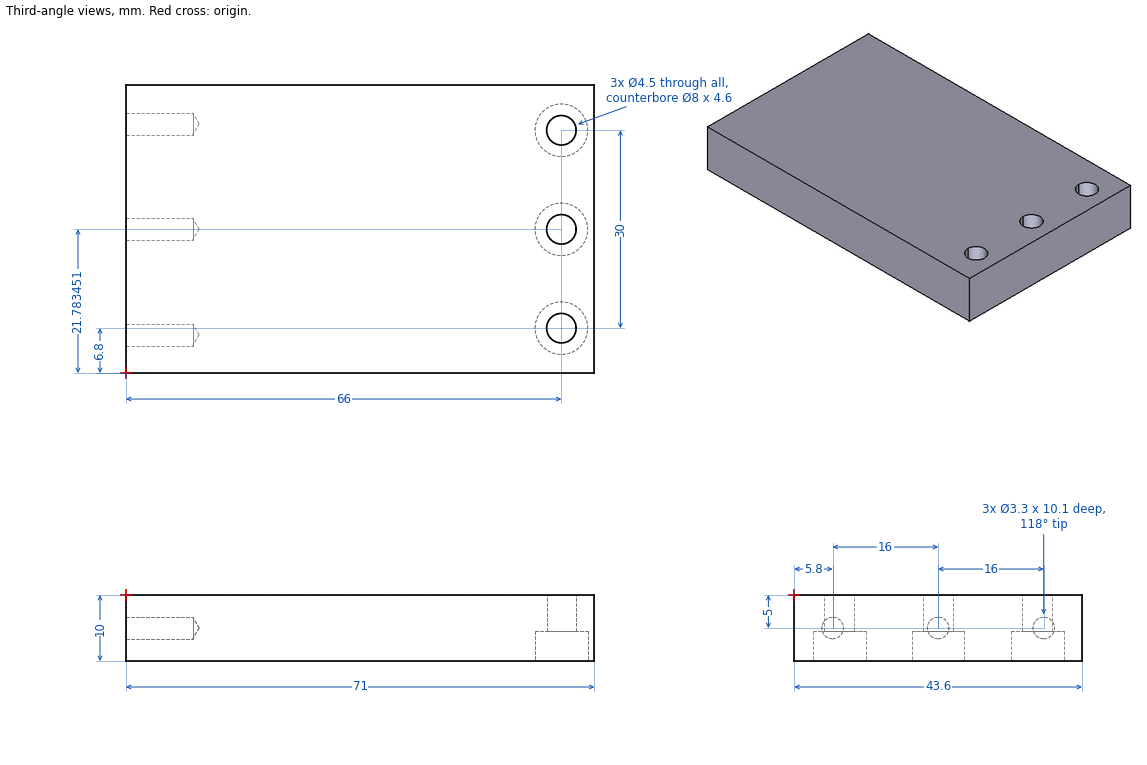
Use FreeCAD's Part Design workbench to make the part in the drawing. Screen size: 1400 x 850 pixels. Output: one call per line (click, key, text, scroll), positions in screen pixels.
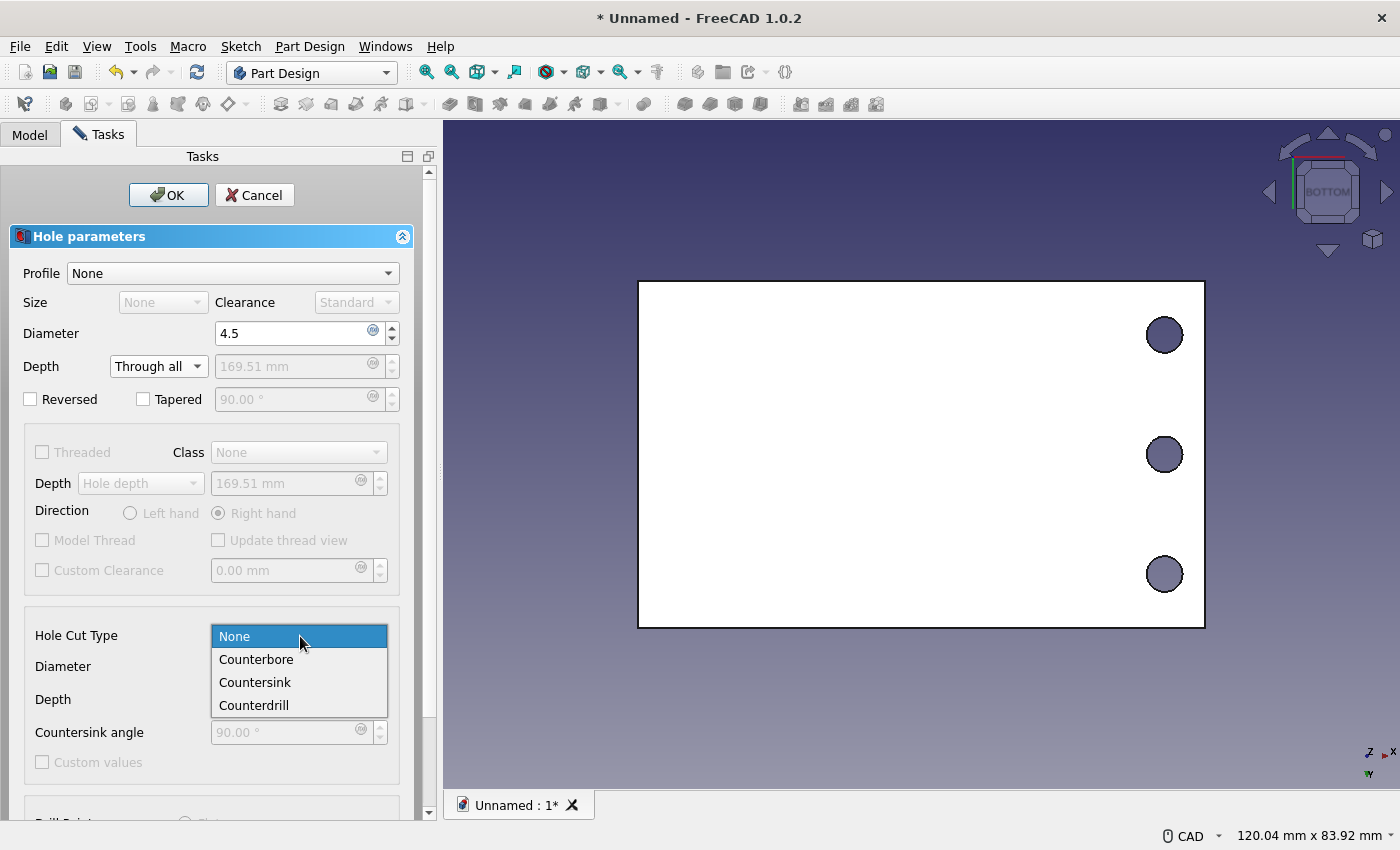
click(298, 660)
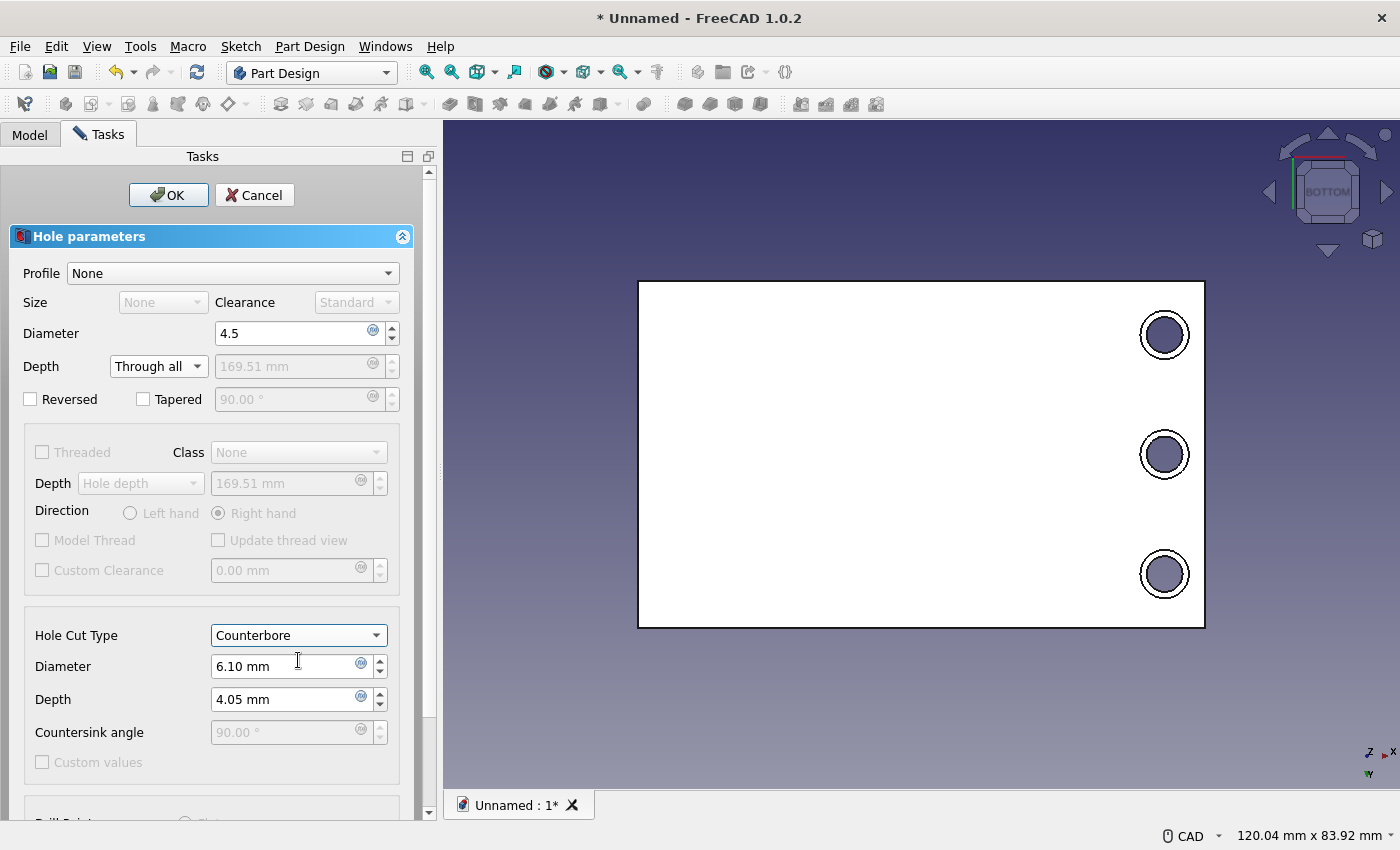
triple_click(292, 666)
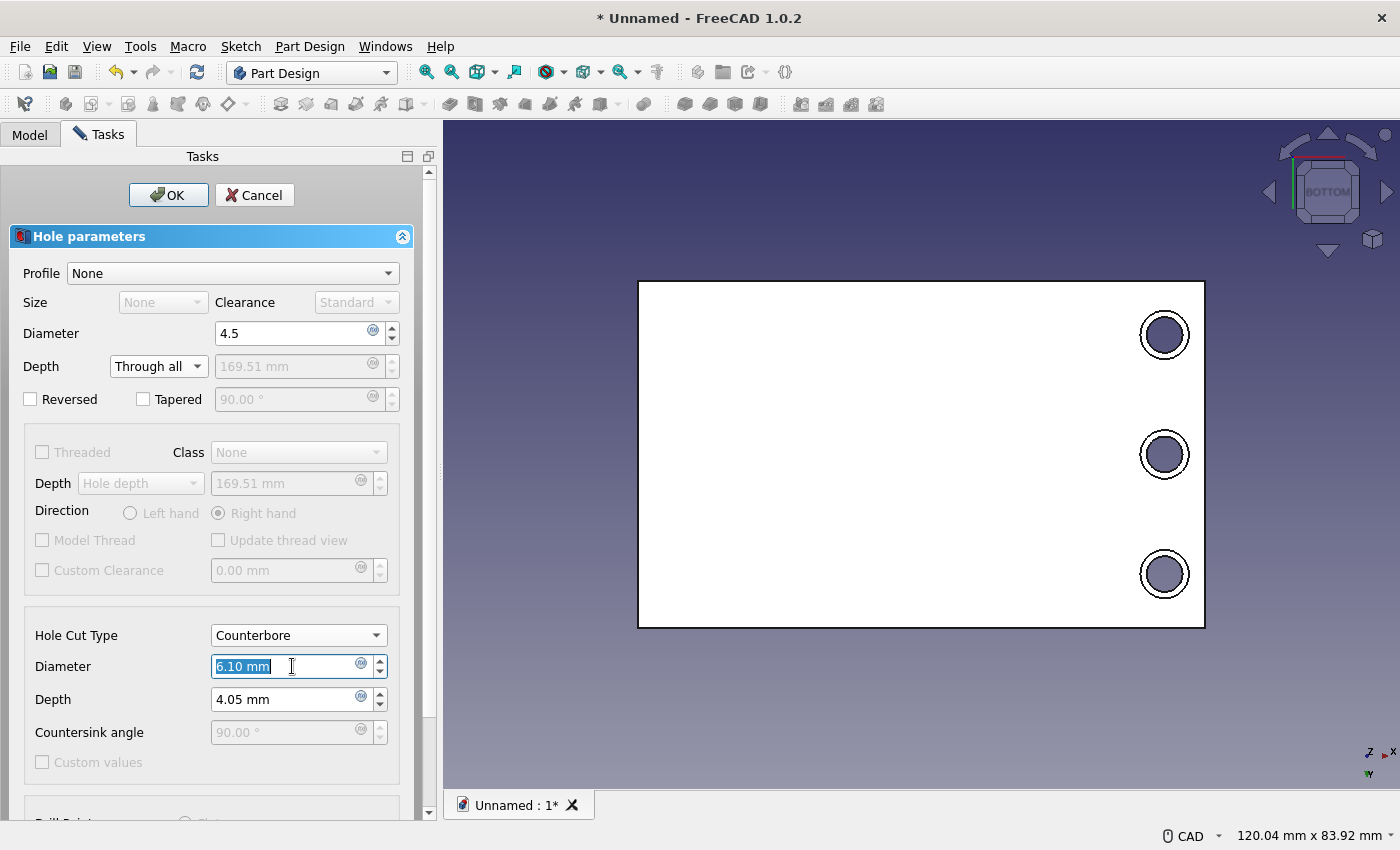
text(8)
key(Tab)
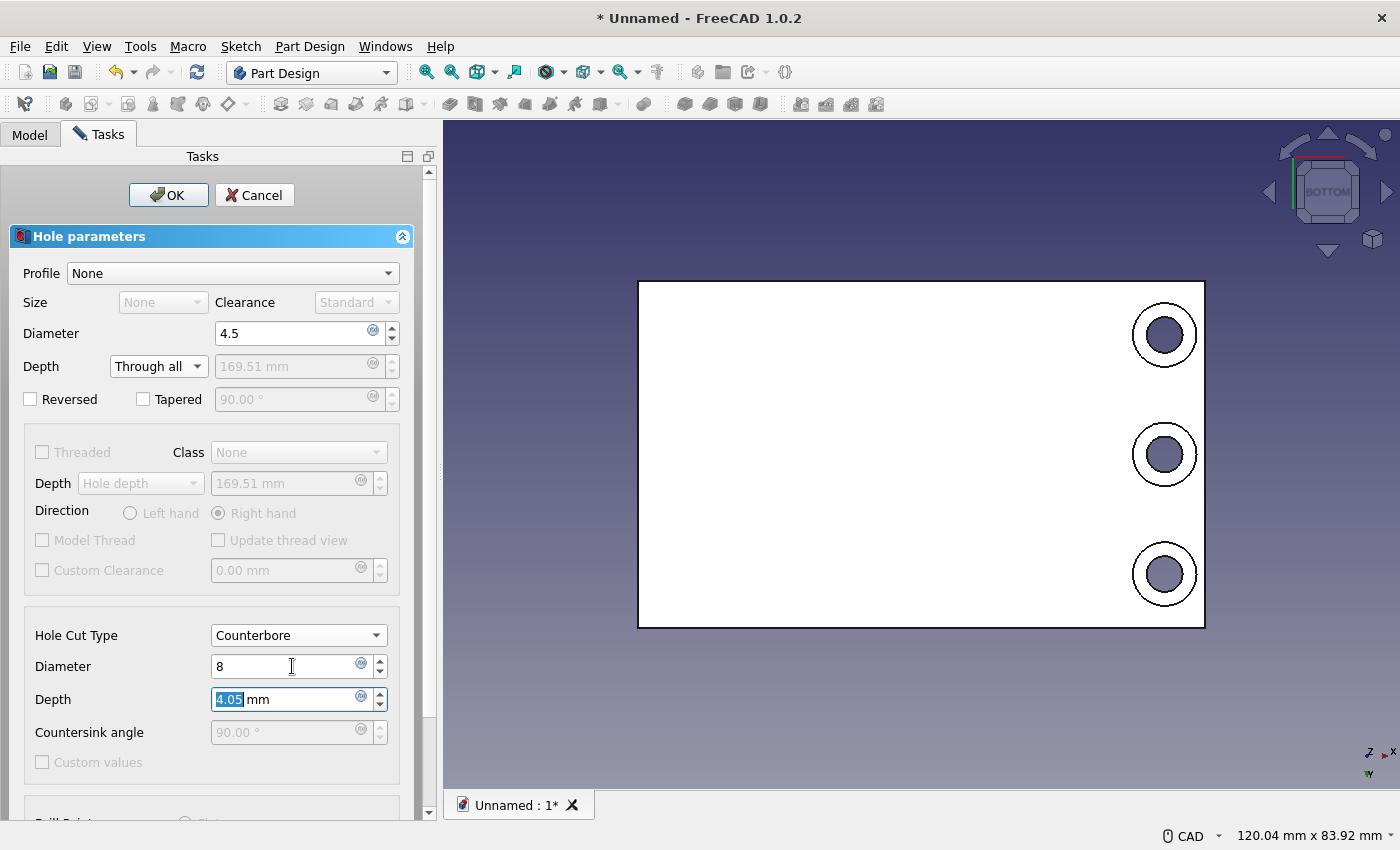
text(4.6)
key(Tab)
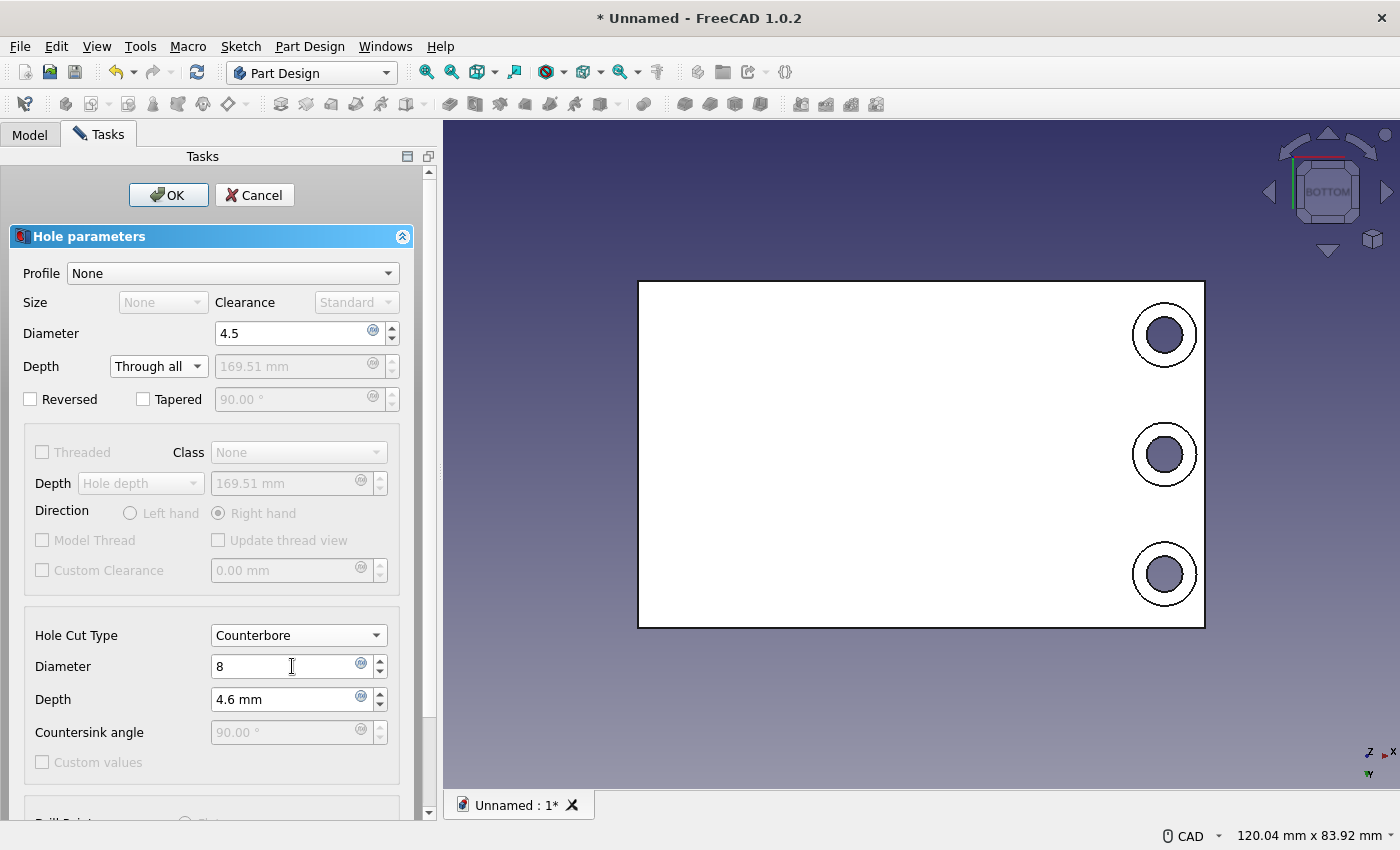
click(169, 195)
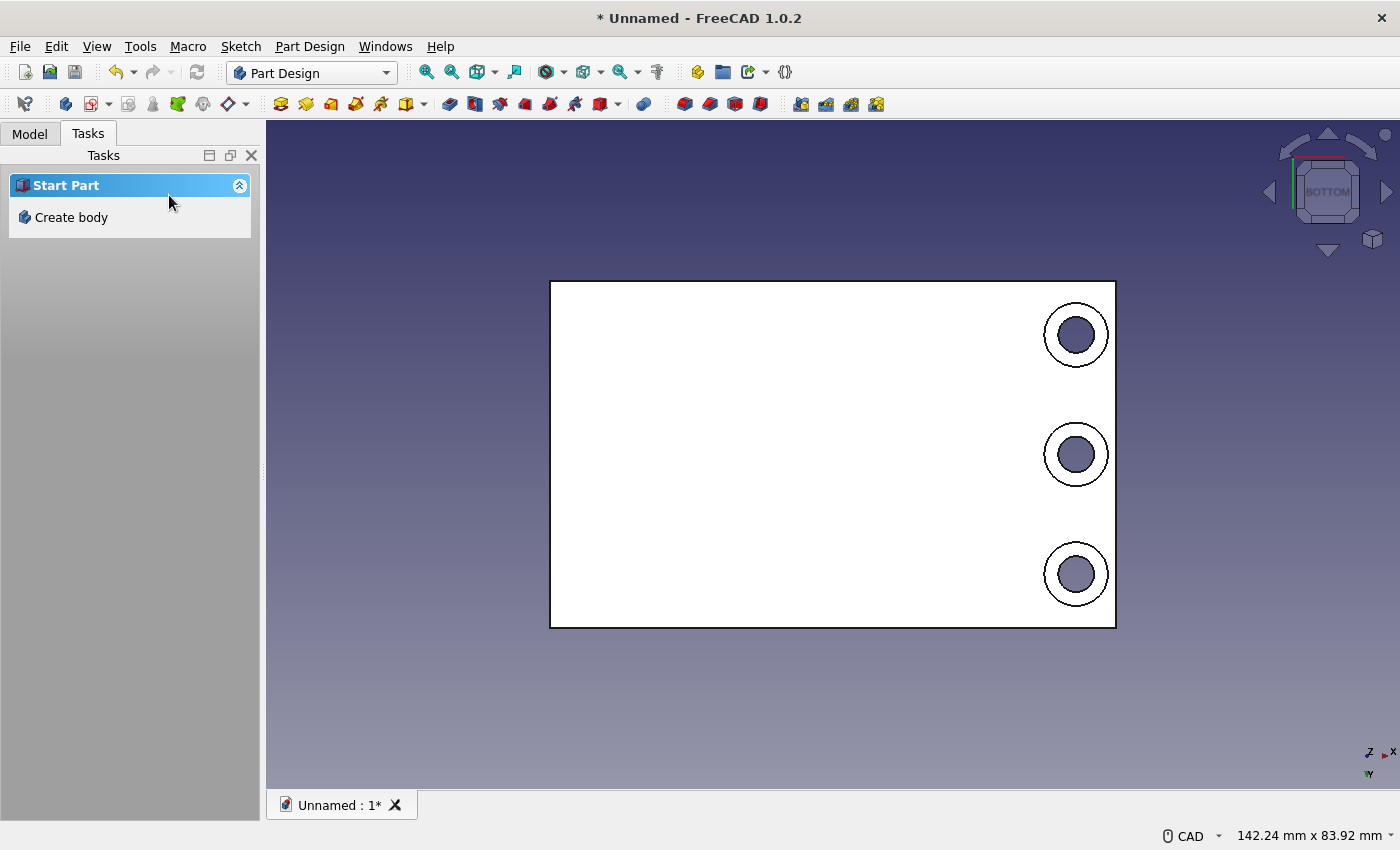
click(90, 104)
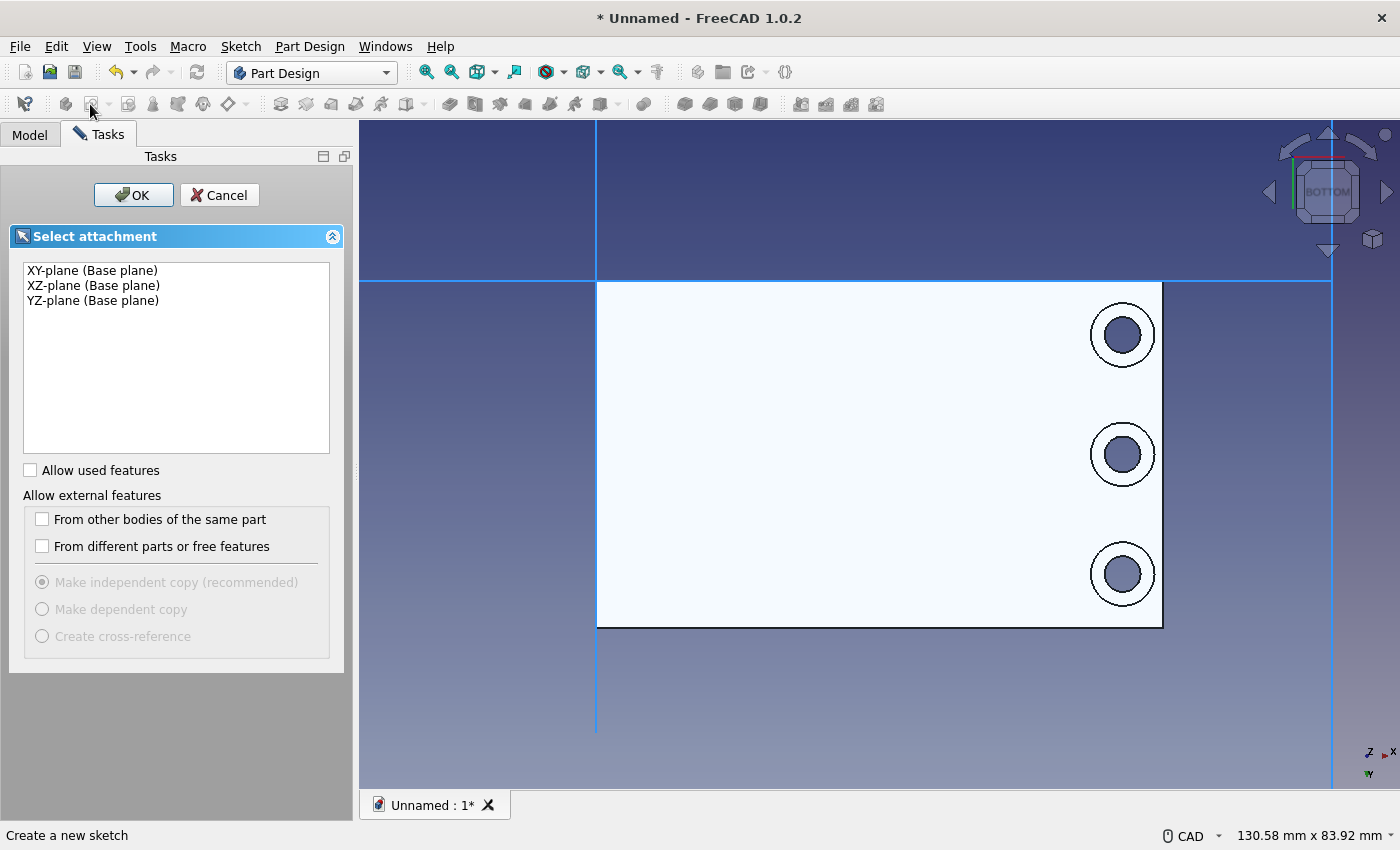
click(84, 300)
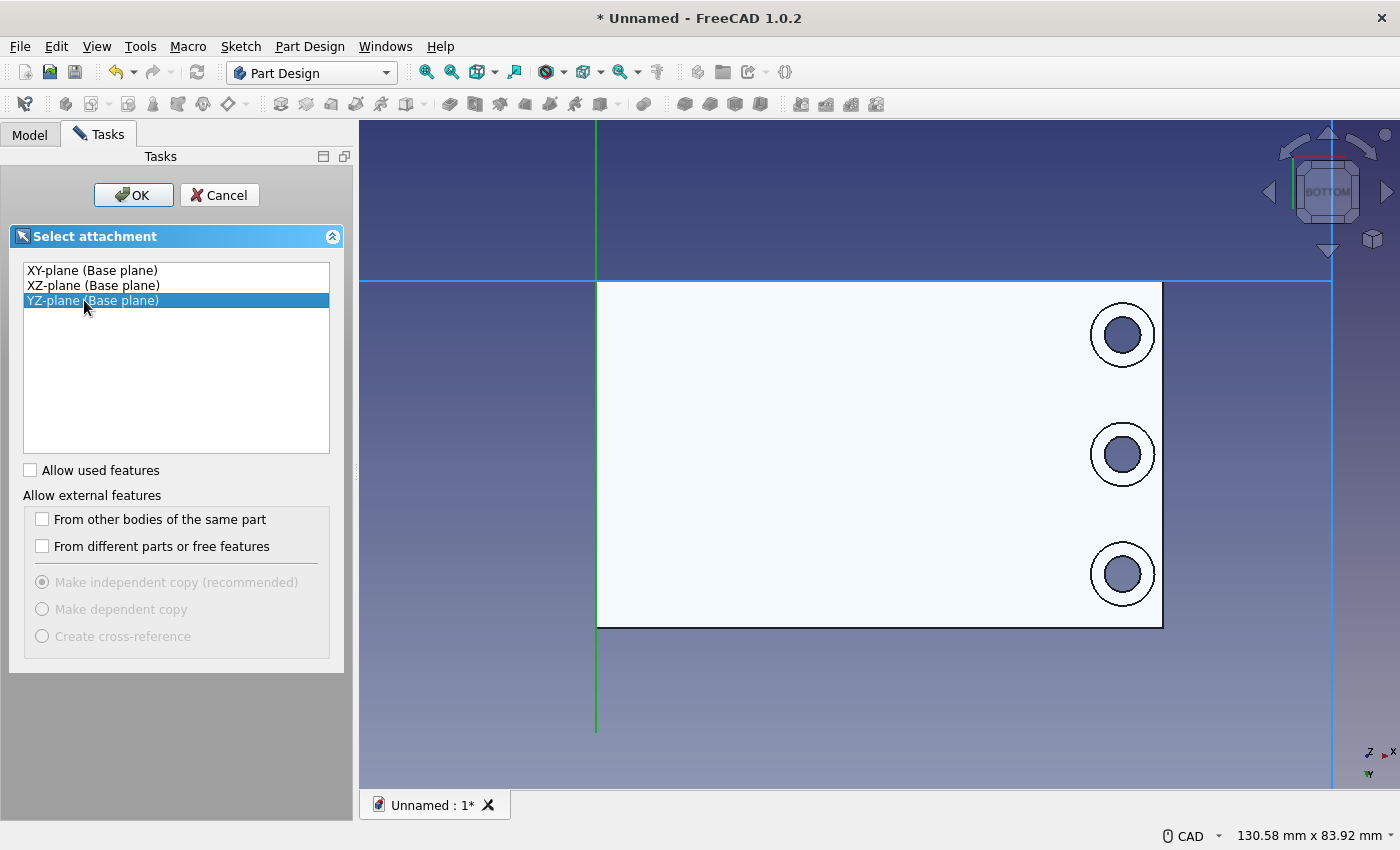
click(134, 195)